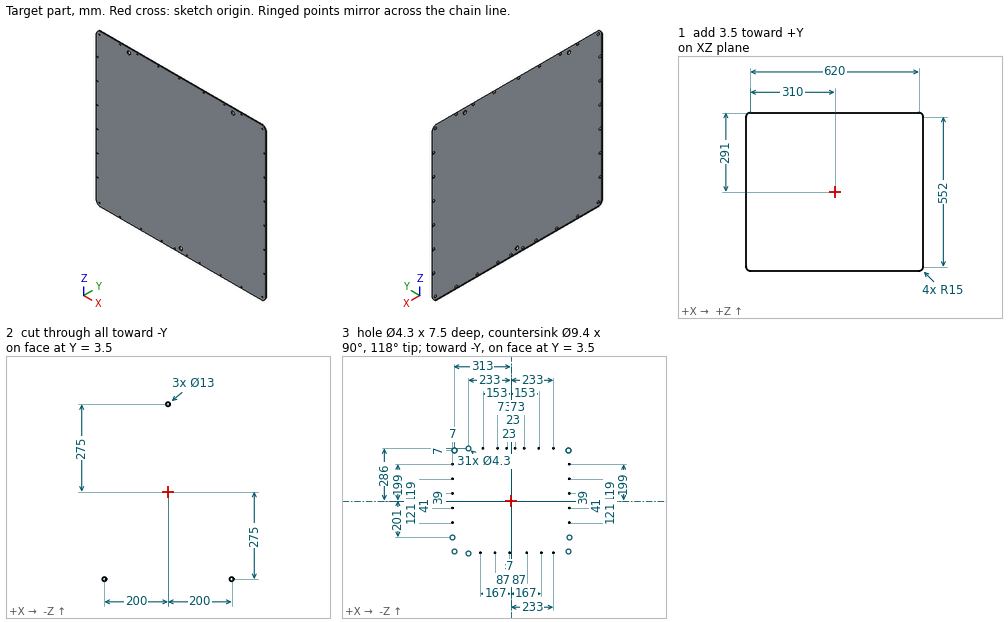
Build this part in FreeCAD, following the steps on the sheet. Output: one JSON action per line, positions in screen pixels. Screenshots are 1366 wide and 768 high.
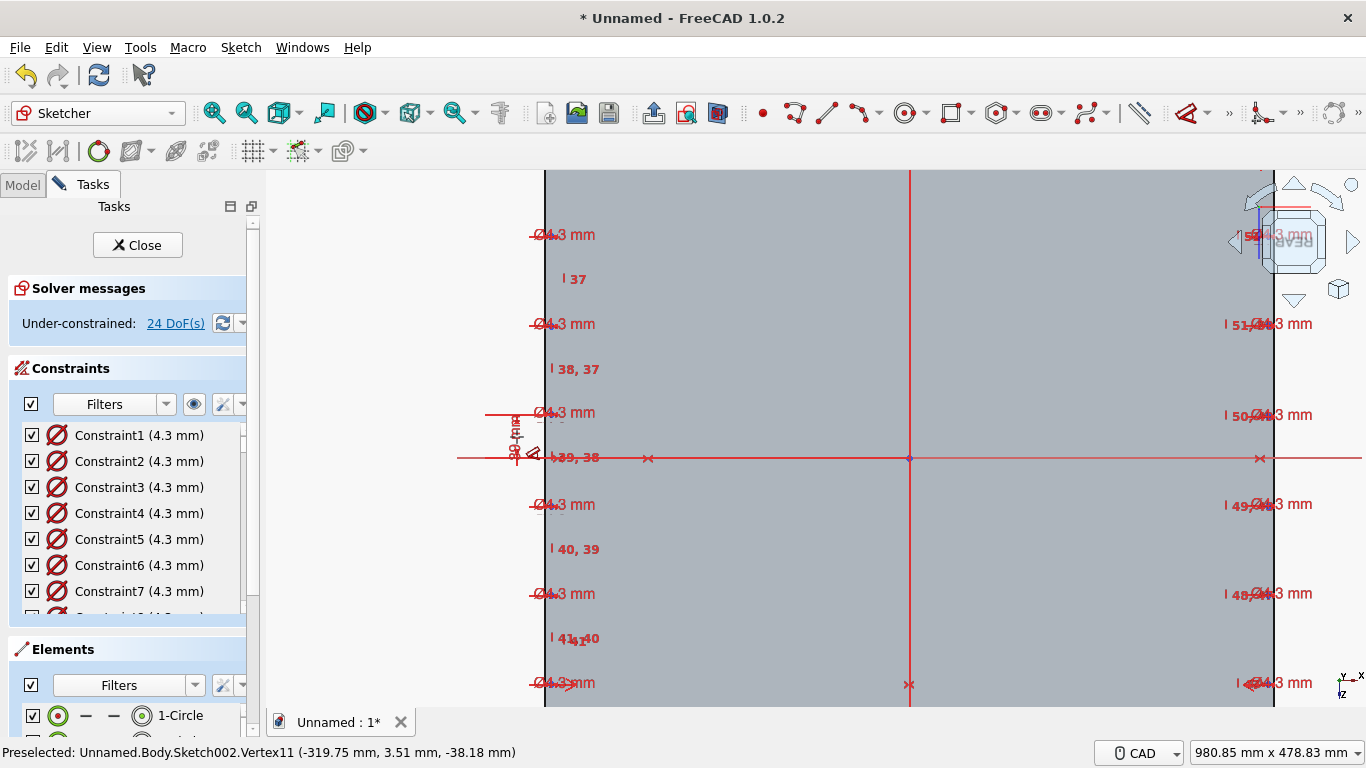
{"action": "left_click", "coordinate": [551, 507]}
{"action": "left_click", "coordinate": [517, 482]}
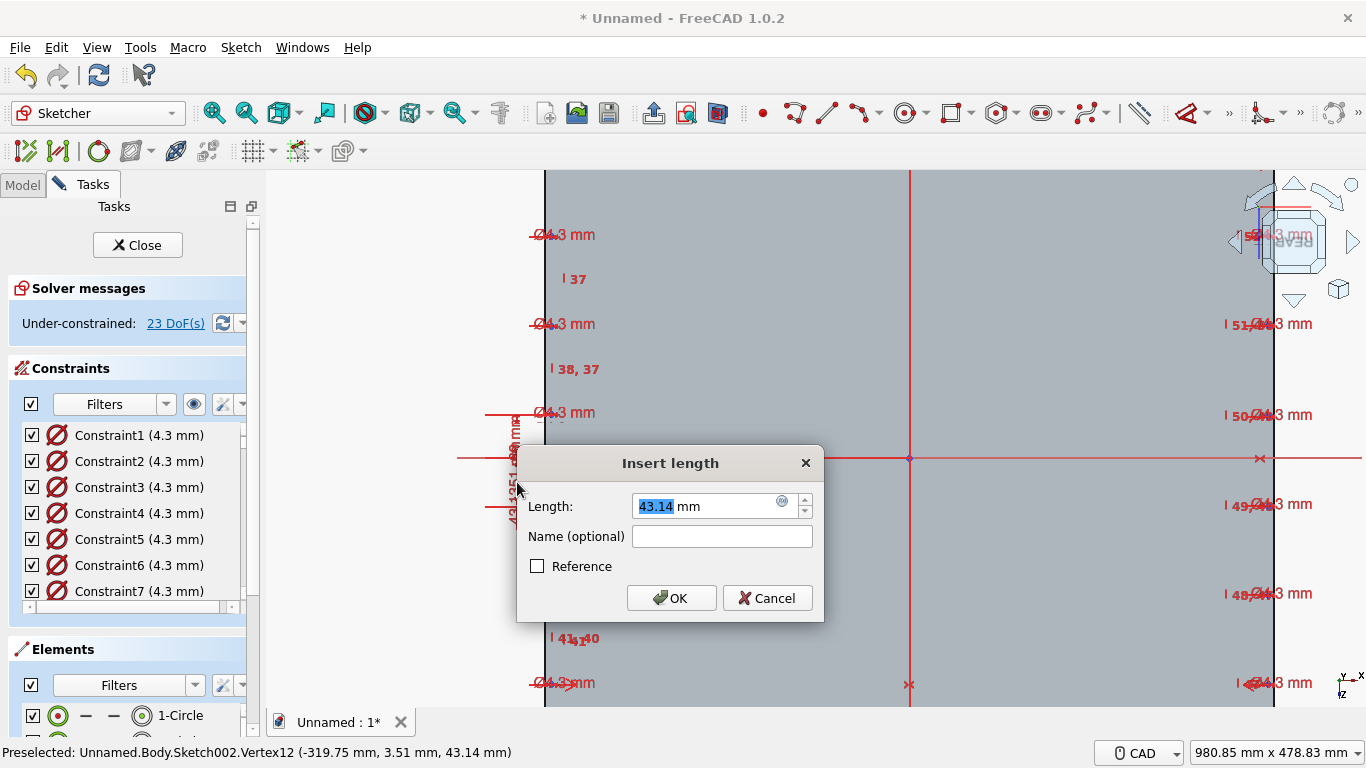
{"action": "type", "text": "41"}
{"action": "key", "text": "Return"}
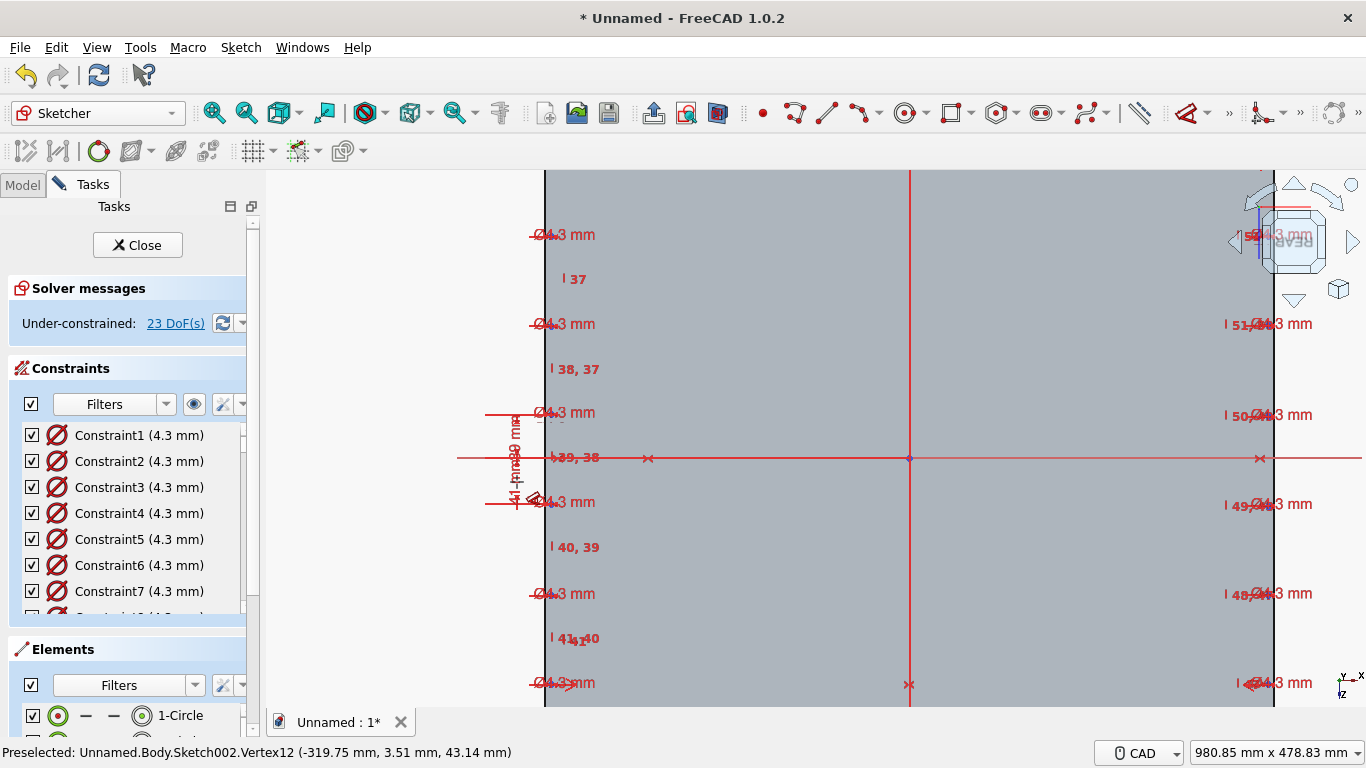
{"action": "scroll", "coordinate": [550, 414], "scroll_direction": "down", "scroll_amount": 3}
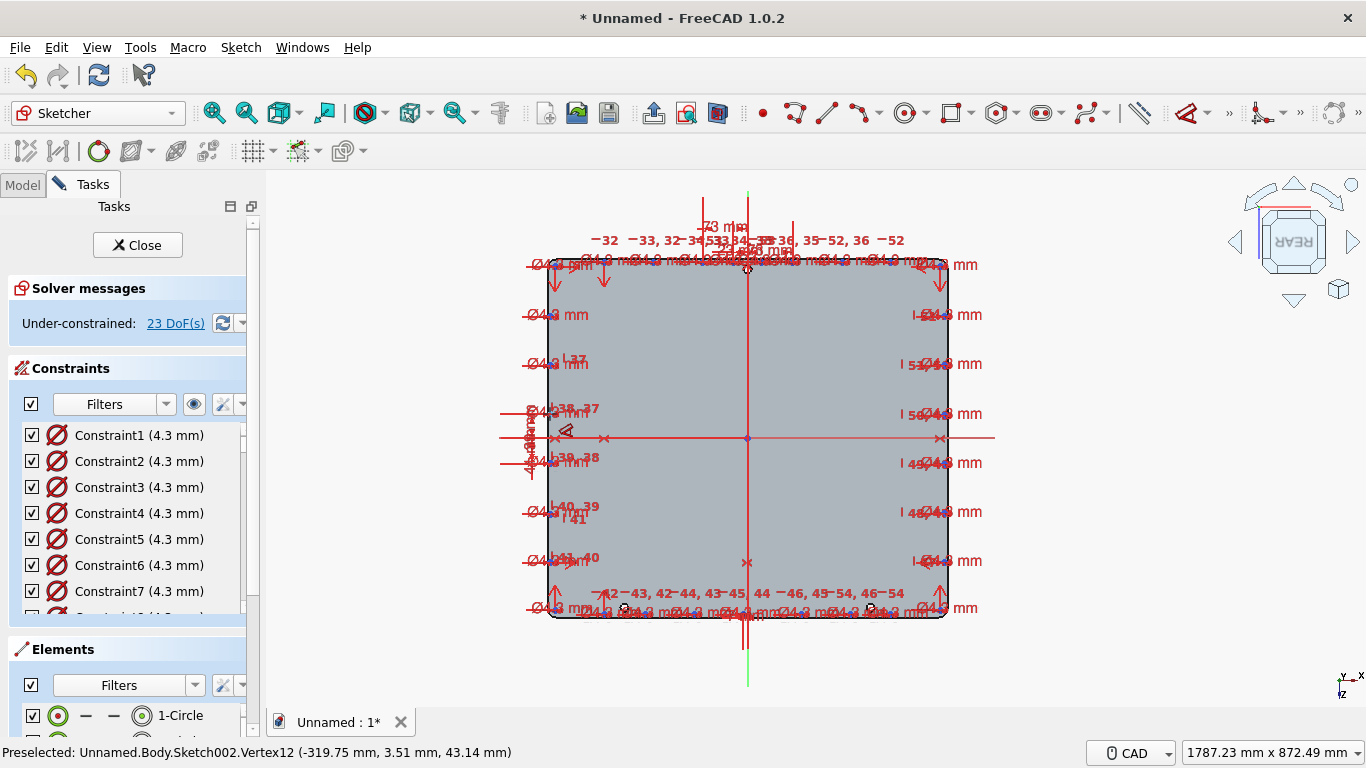
{"action": "left_click", "coordinate": [694, 615]}
{"action": "left_click", "coordinate": [721, 649]}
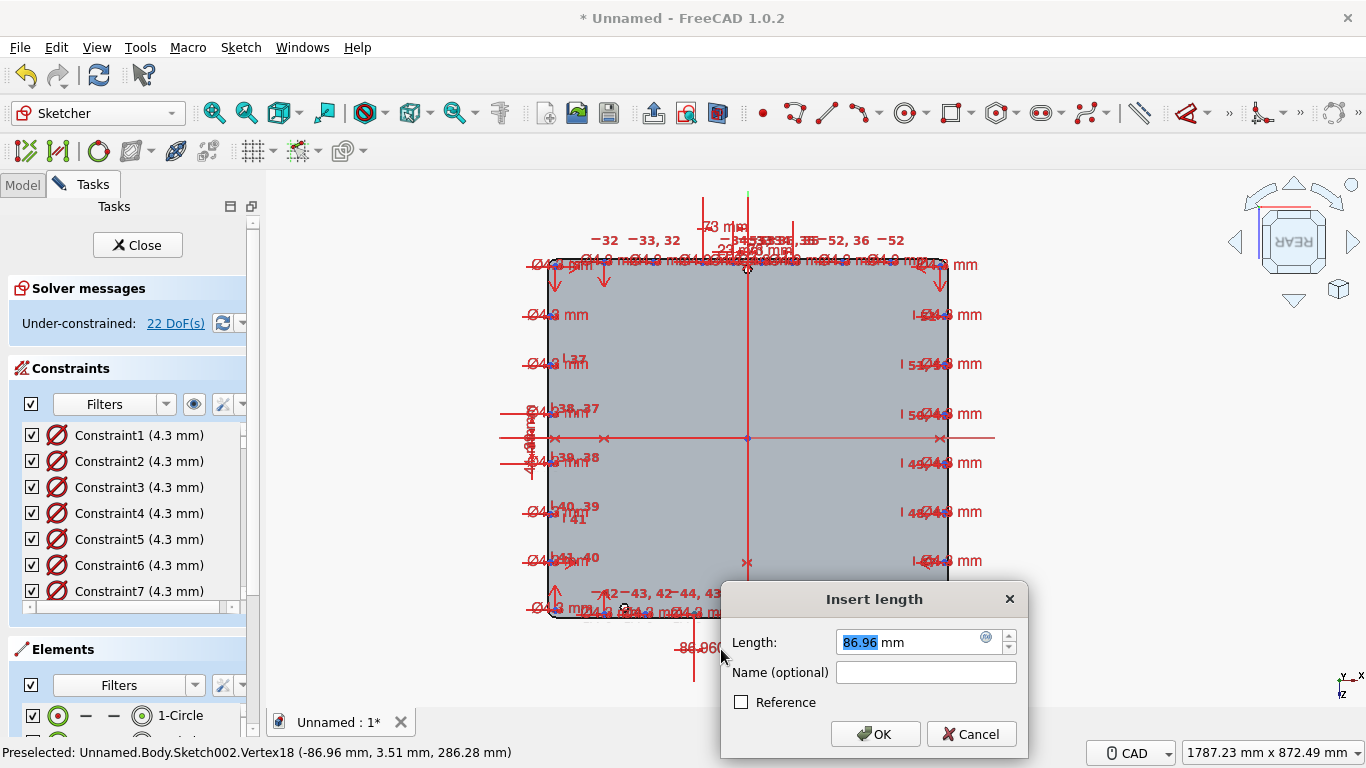
{"action": "type", "text": "87"}
{"action": "key", "text": "Return"}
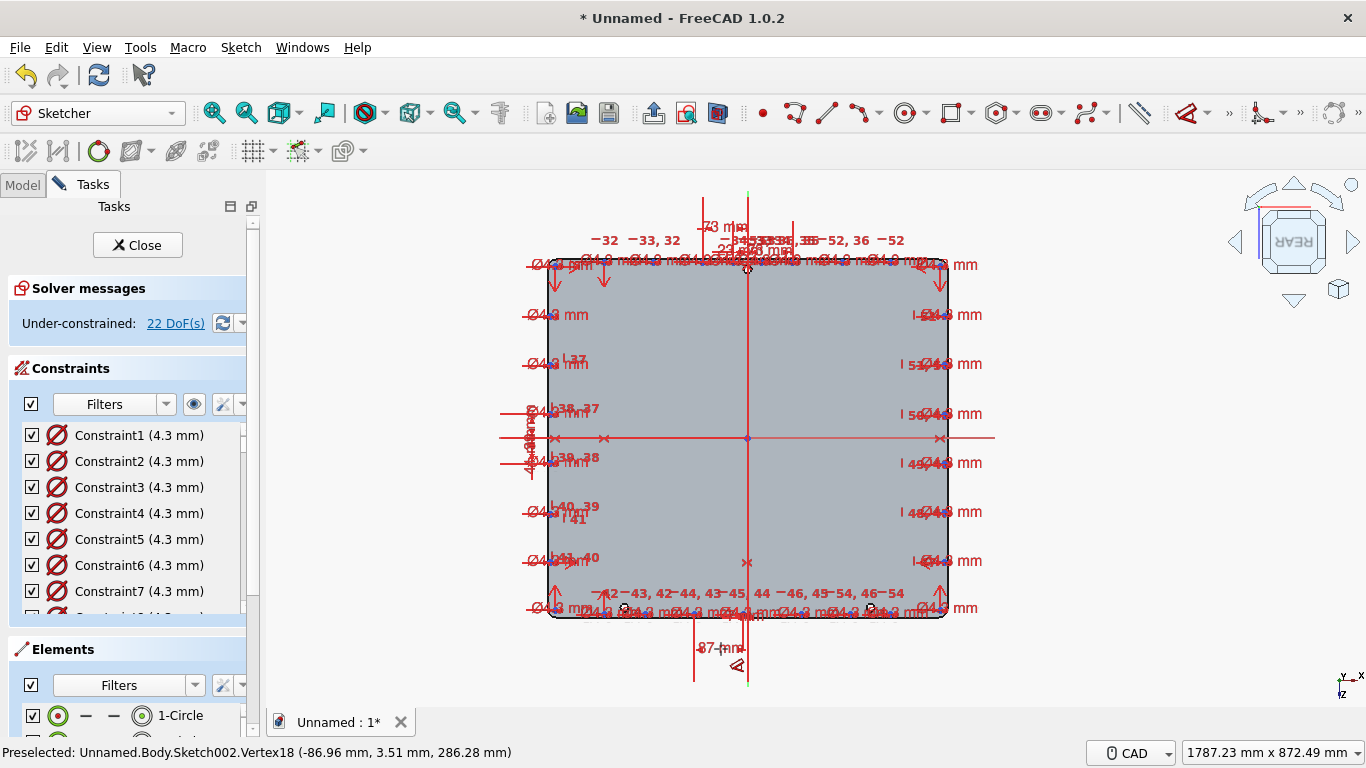
{"action": "left_click", "coordinate": [802, 615]}
{"action": "left_click", "coordinate": [793, 649]}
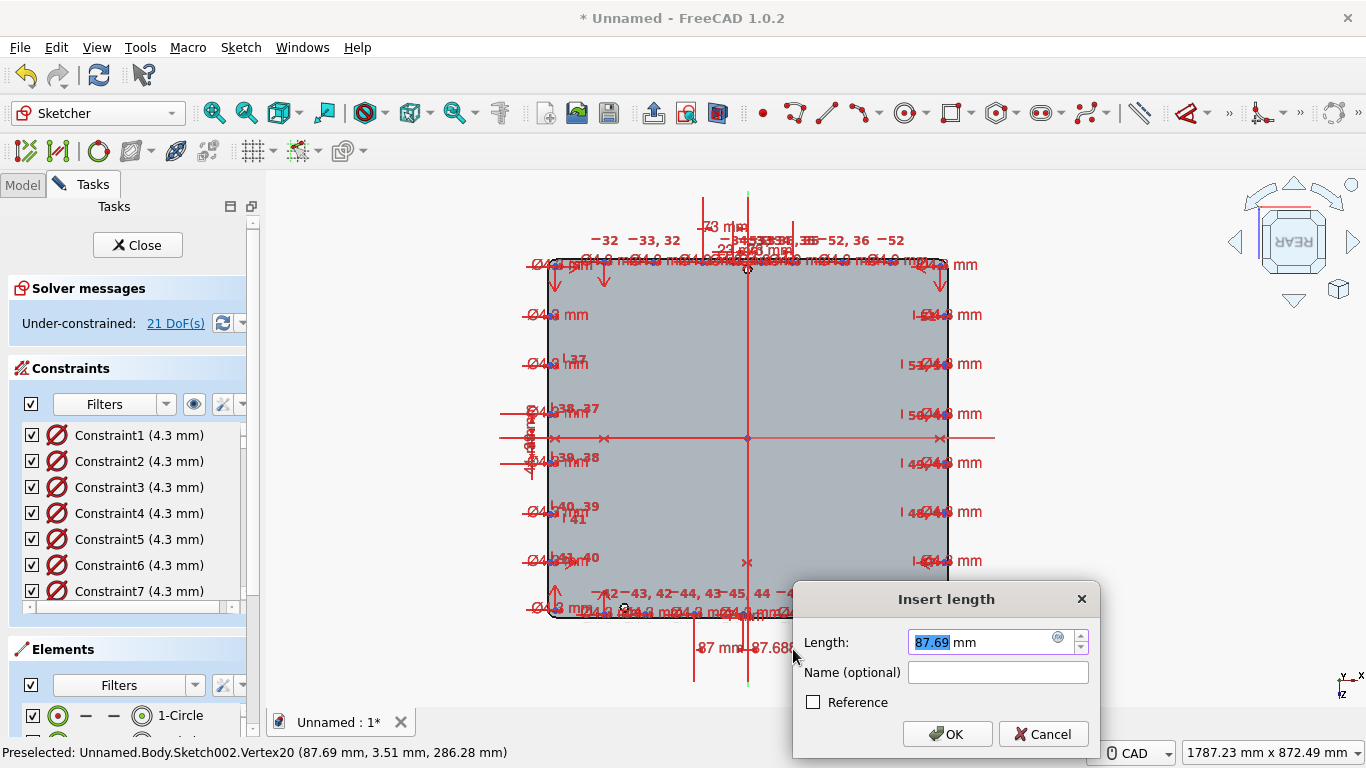
{"action": "type", "text": "87"}
{"action": "key", "text": "Return"}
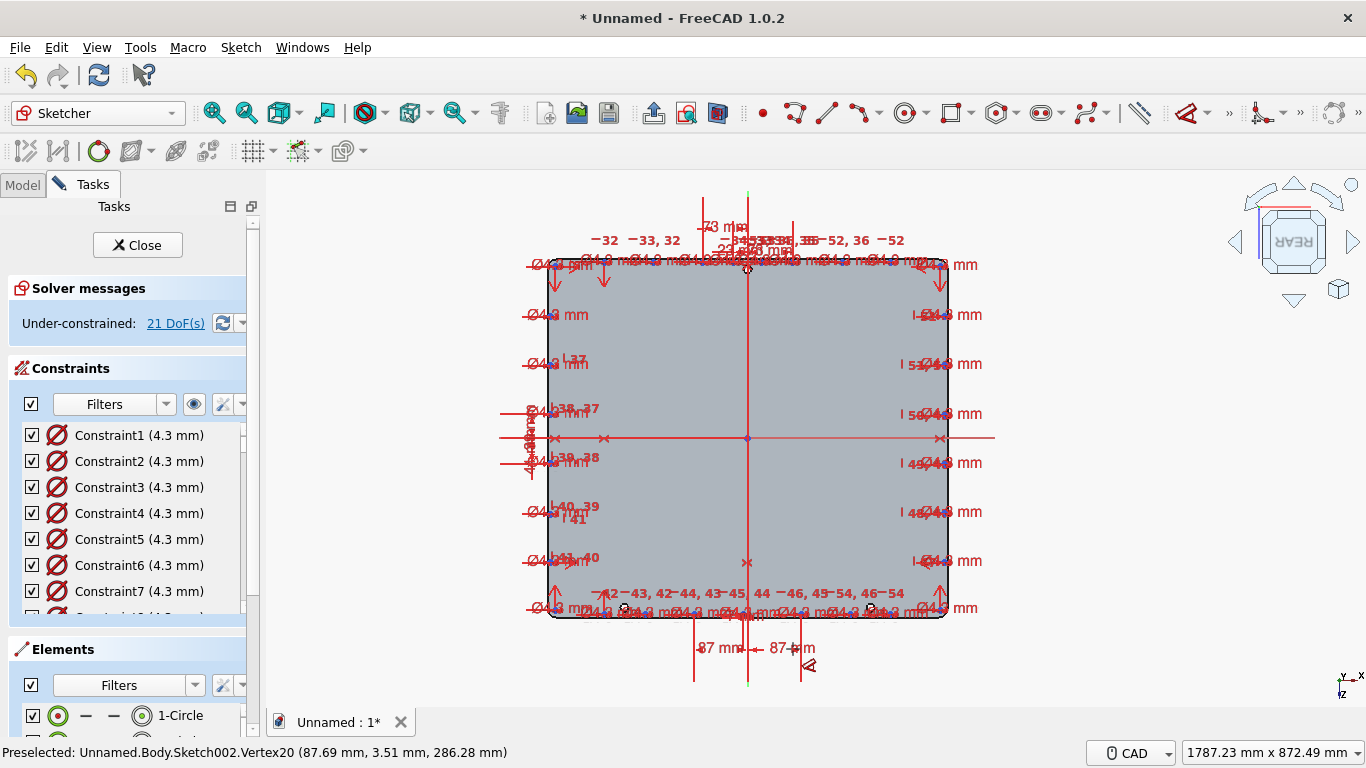
{"action": "scroll", "coordinate": [944, 465], "scroll_direction": "up", "scroll_amount": 3}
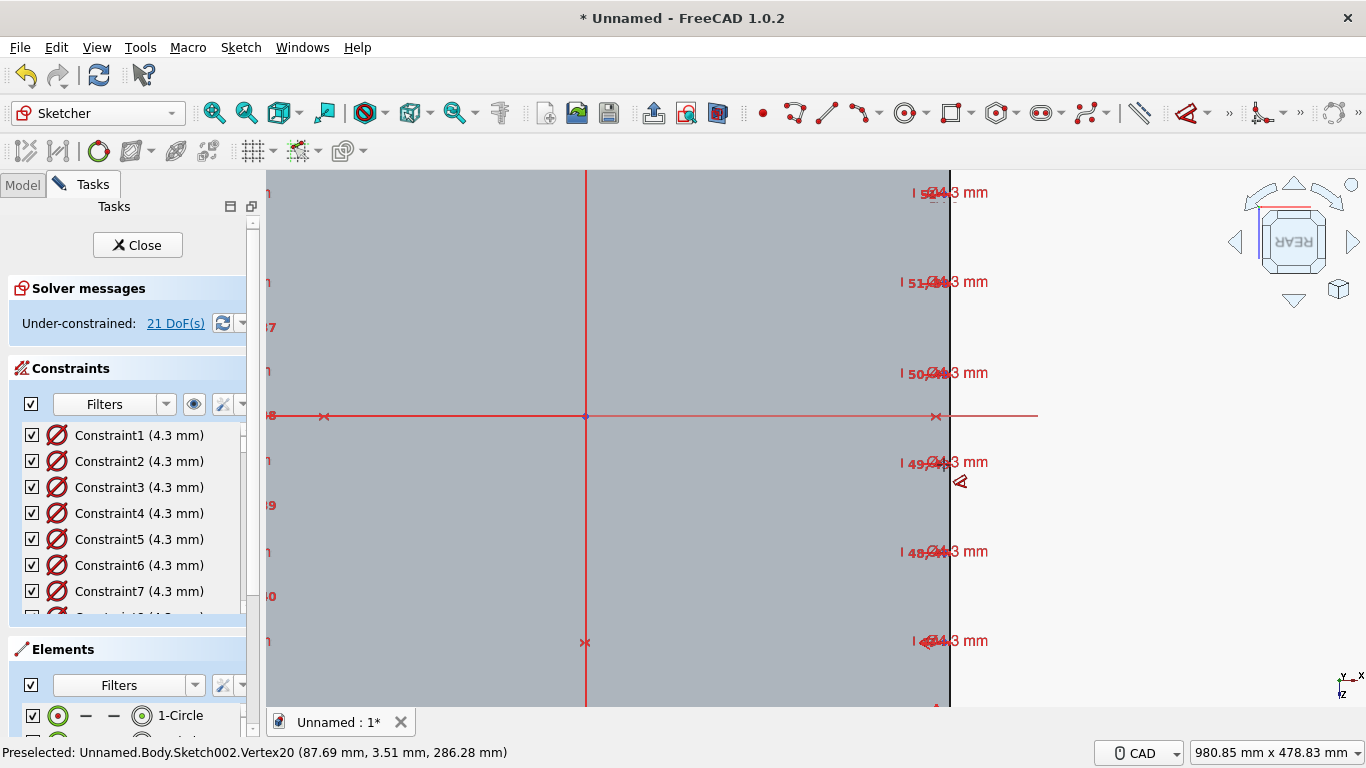
{"action": "left_click", "coordinate": [944, 464]}
{"action": "left_click", "coordinate": [978, 440]}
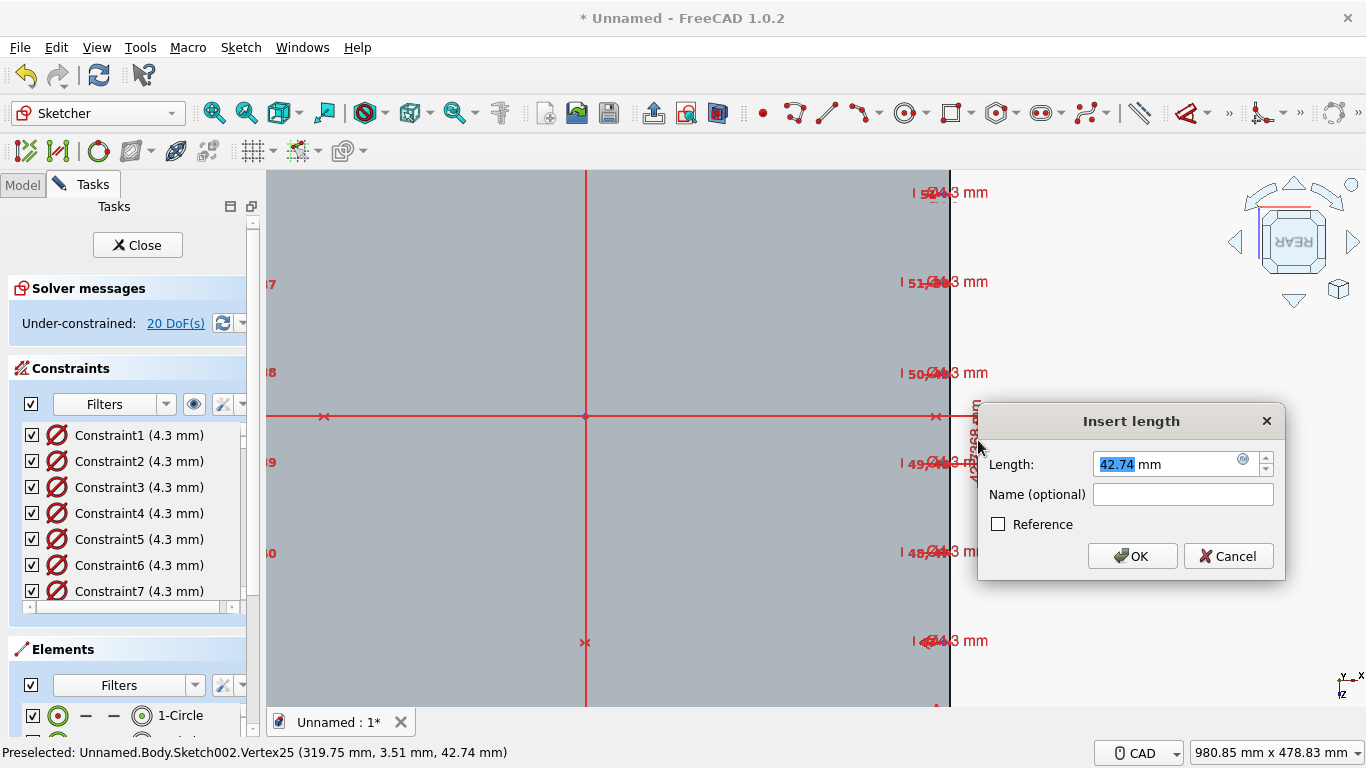
{"action": "type", "text": "41"}
{"action": "key", "text": "Return"}